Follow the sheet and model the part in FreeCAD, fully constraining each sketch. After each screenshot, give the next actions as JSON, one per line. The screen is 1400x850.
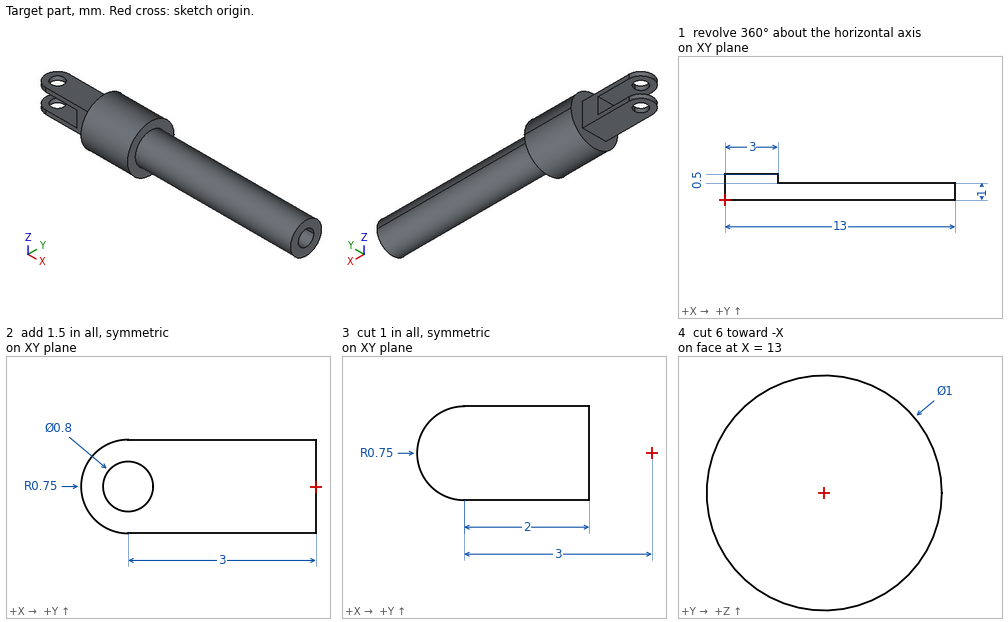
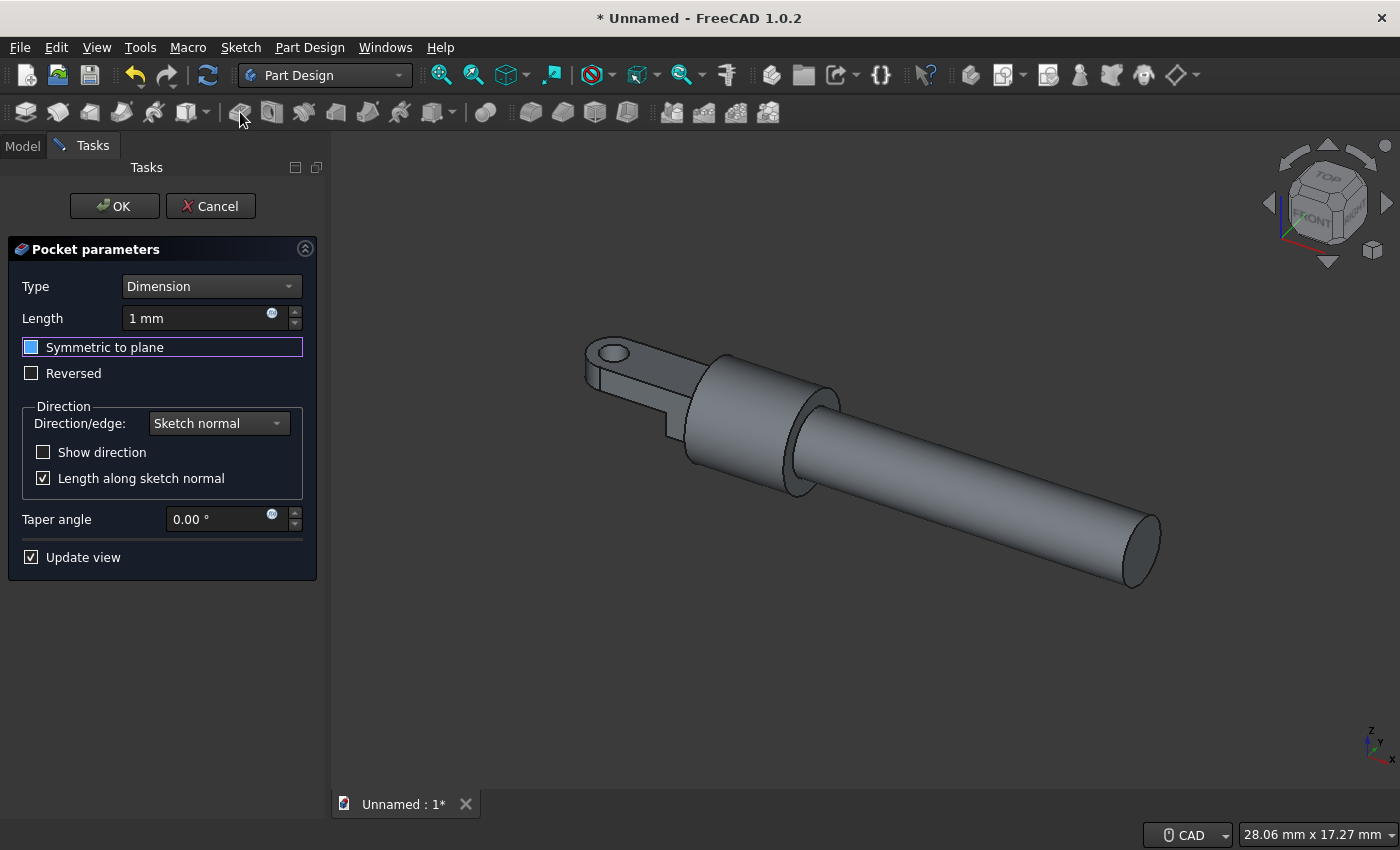
{"action": "left_click", "coordinate": [30, 347]}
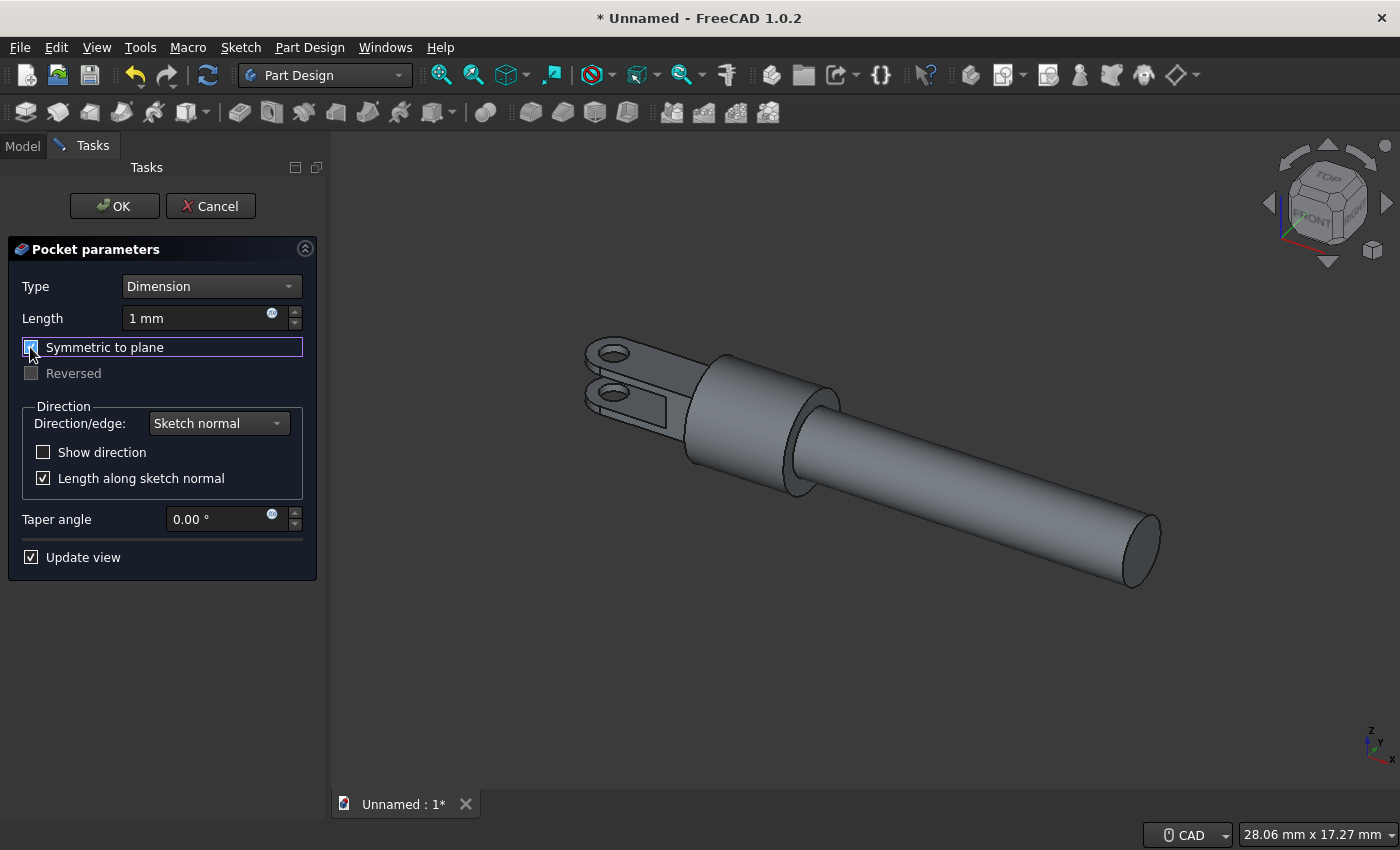
{"action": "left_click", "coordinate": [115, 206]}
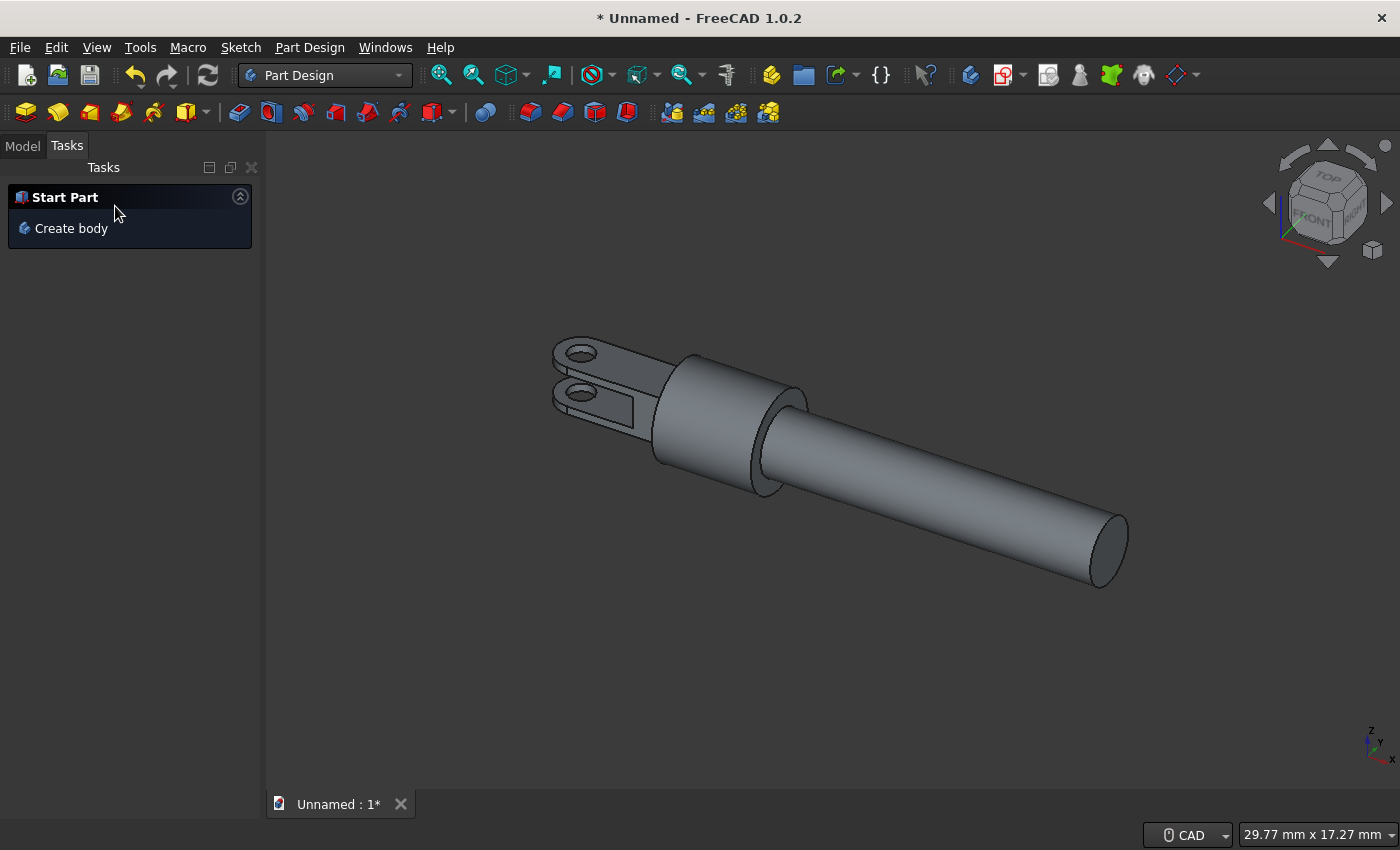
{"action": "left_click", "coordinate": [1109, 550]}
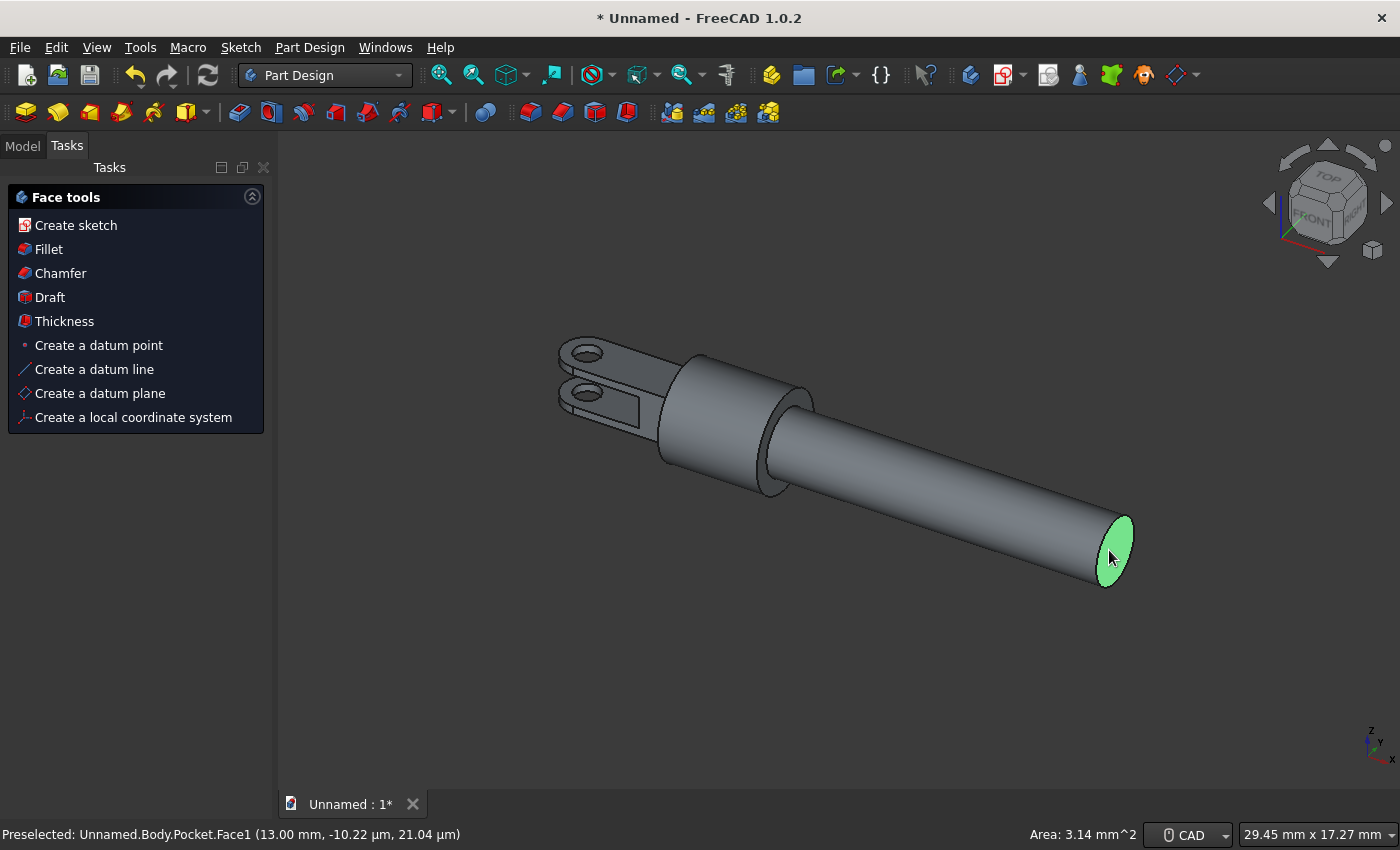
{"action": "left_click", "coordinate": [1004, 76]}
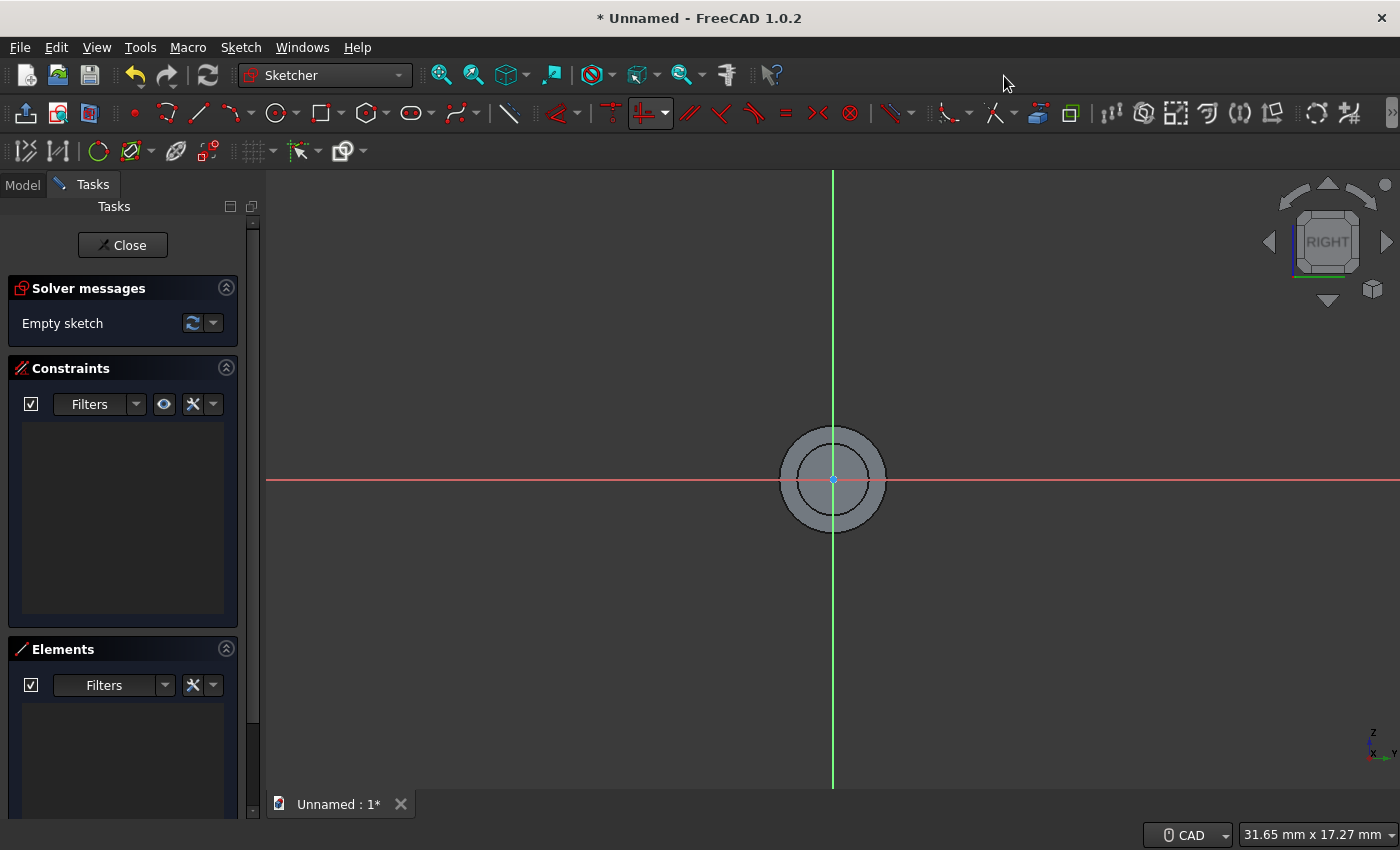
{"action": "scroll", "coordinate": [840, 480], "scroll_direction": "up", "scroll_amount": 12}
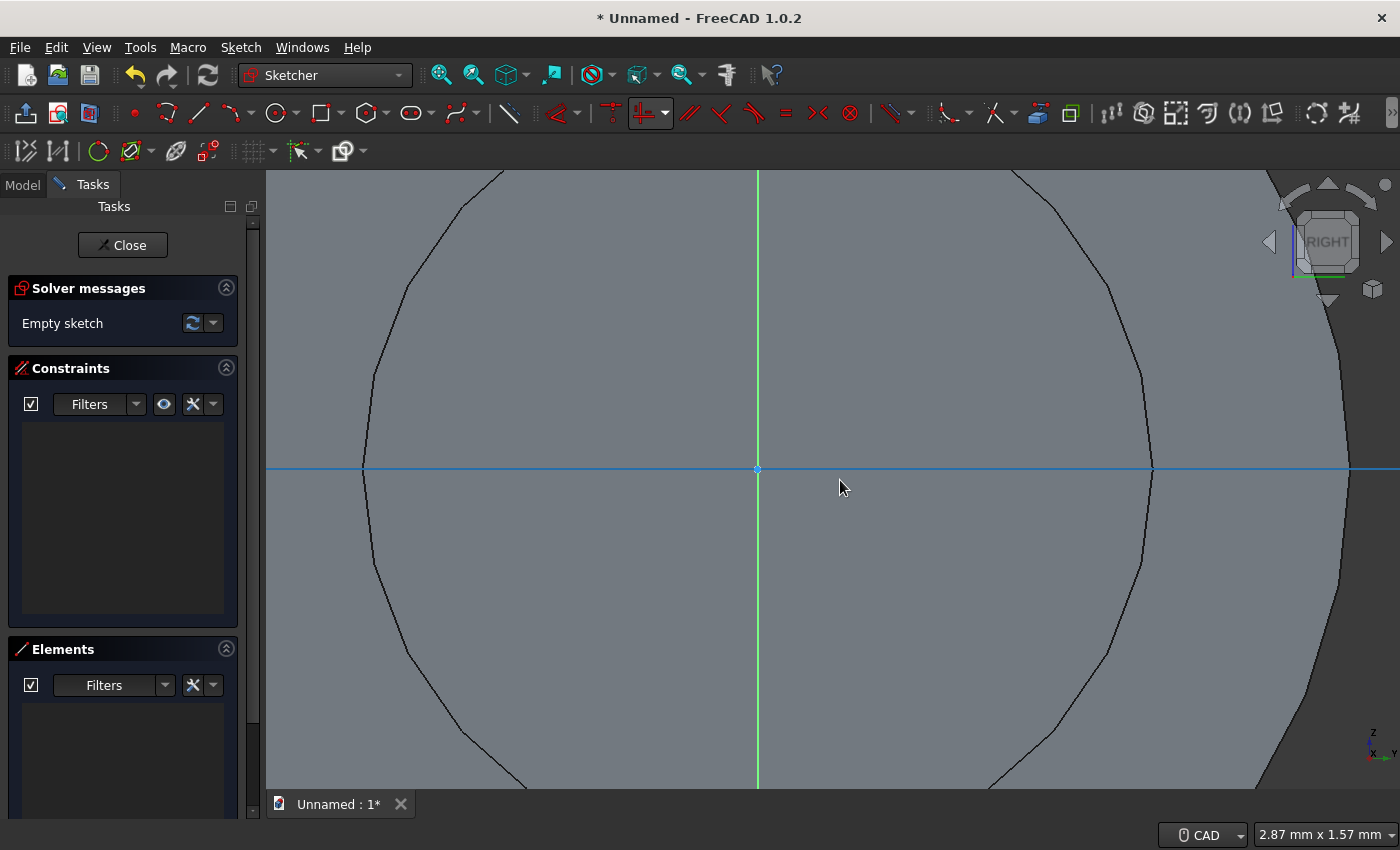
{"action": "key", "text": "g c"}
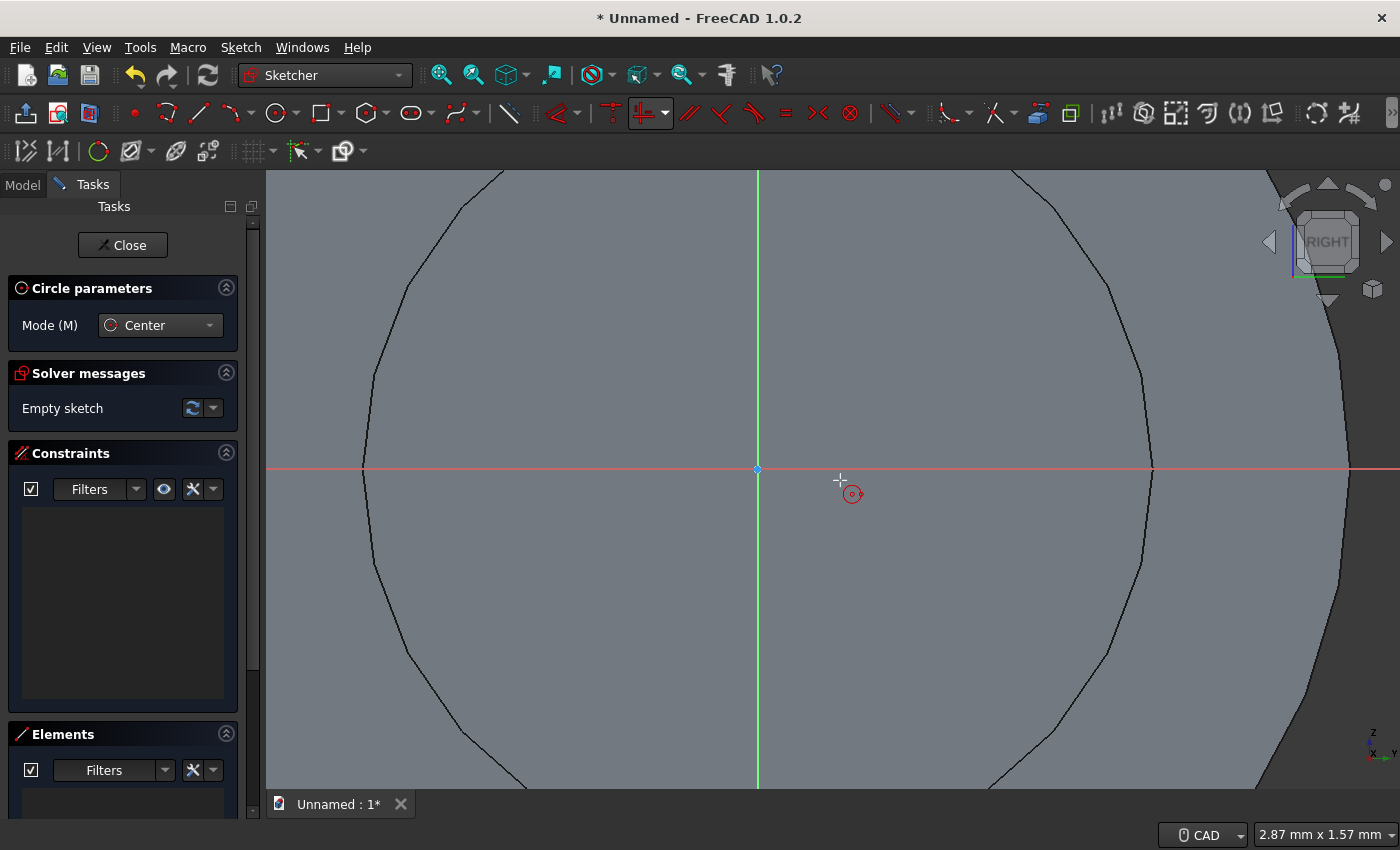
{"action": "left_click", "coordinate": [758, 469]}
{"action": "left_click", "coordinate": [897, 330]}
{"action": "key", "text": "Escape"}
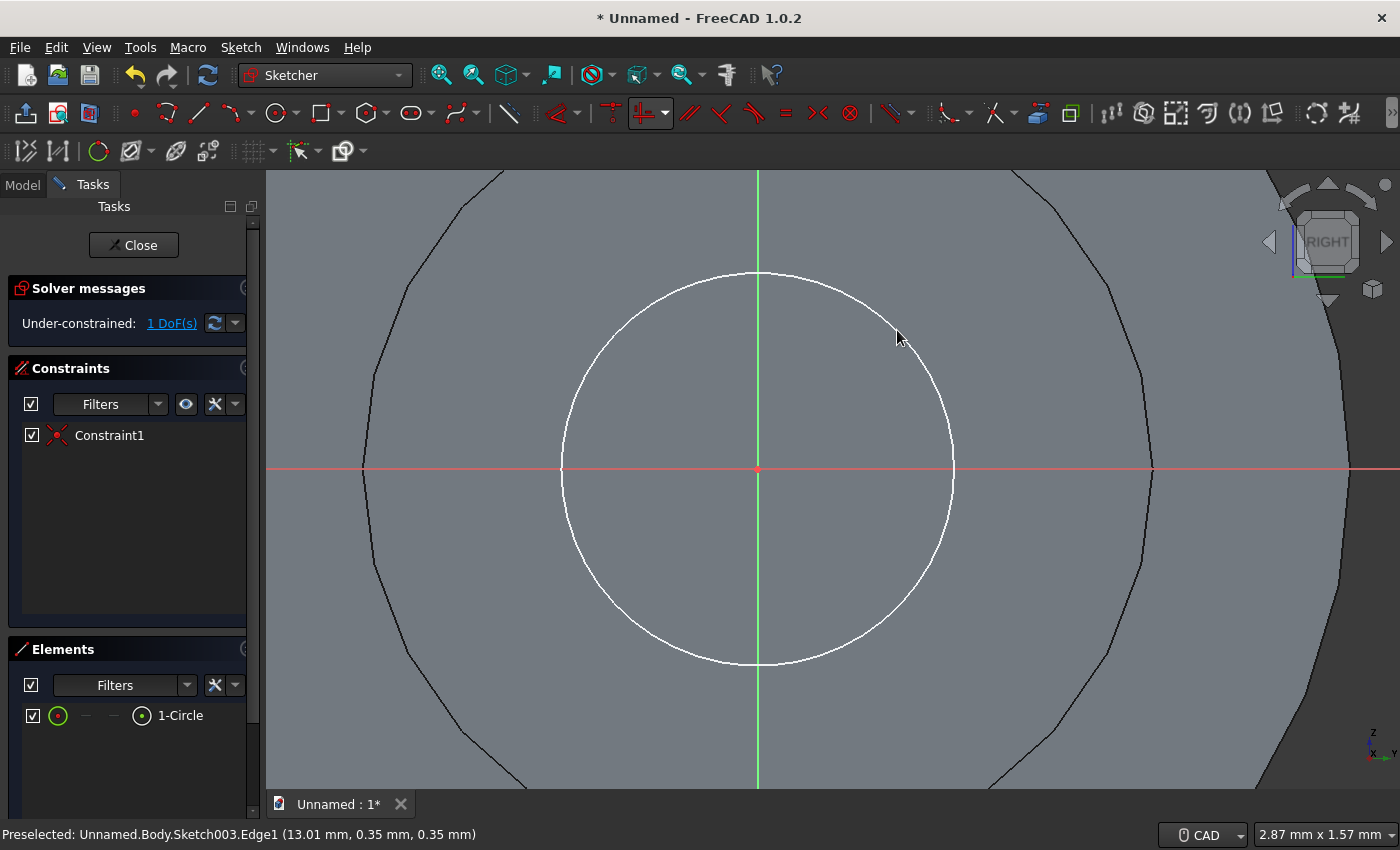
{"action": "left_click", "coordinate": [556, 114]}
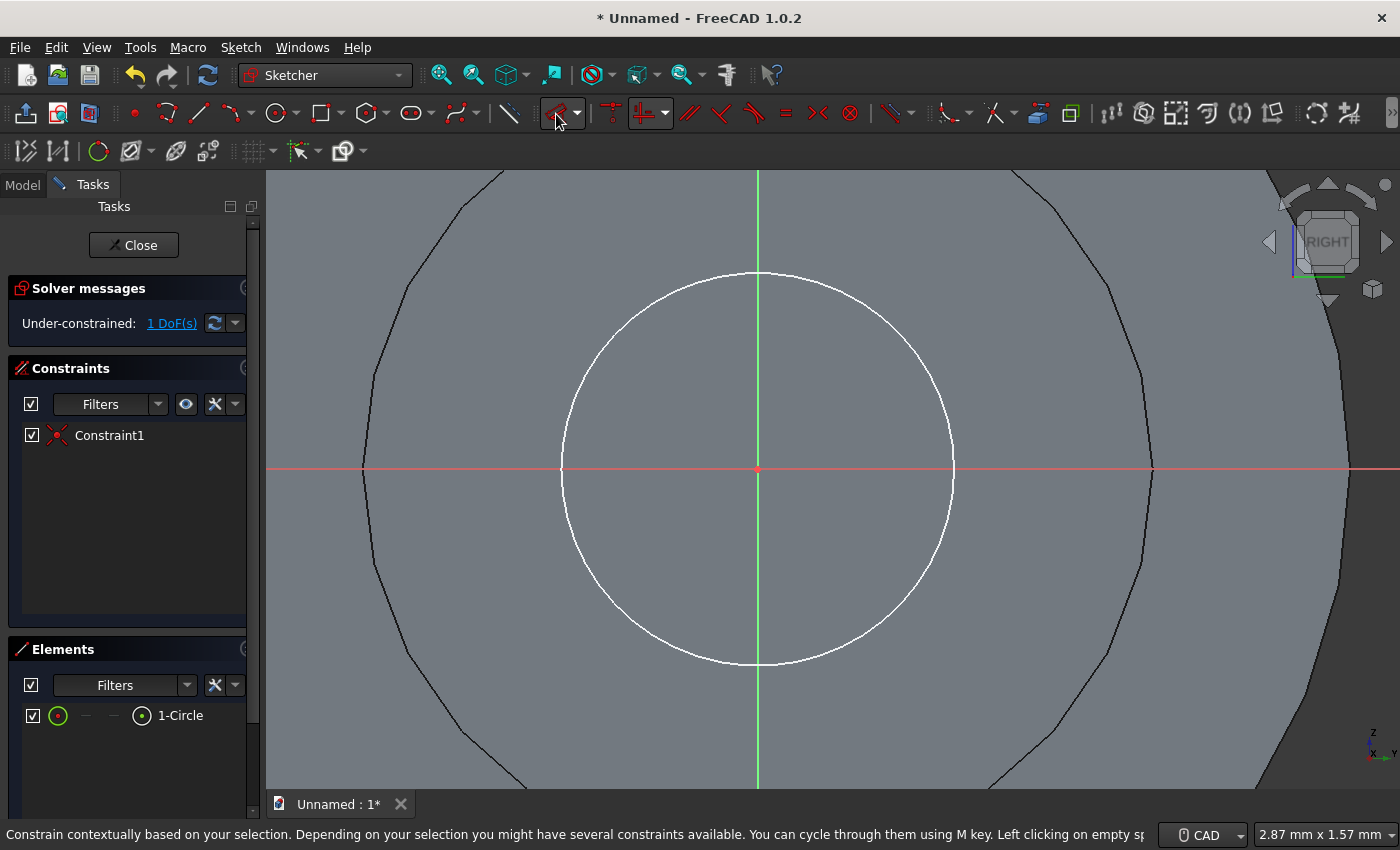
{"action": "left_click", "coordinate": [896, 330]}
{"action": "left_click", "coordinate": [919, 307]}